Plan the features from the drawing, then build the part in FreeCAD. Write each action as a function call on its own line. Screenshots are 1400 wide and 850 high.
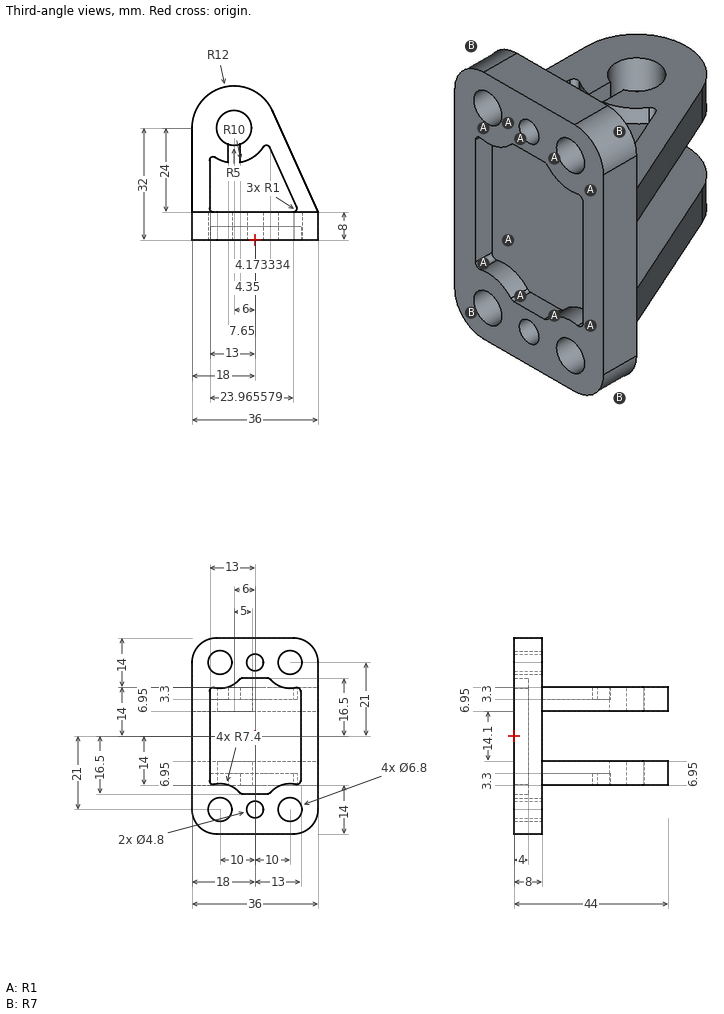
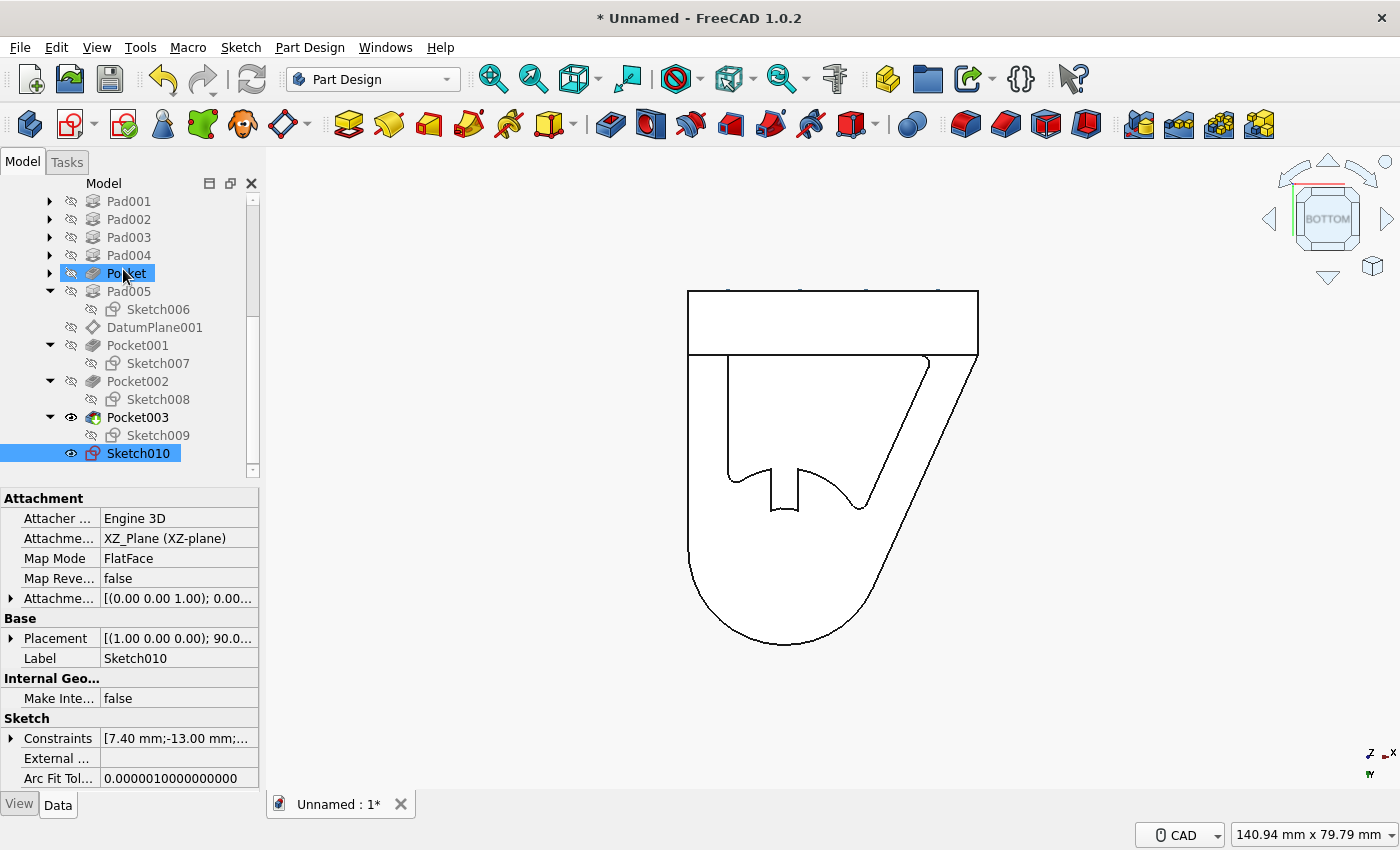
click(612, 124)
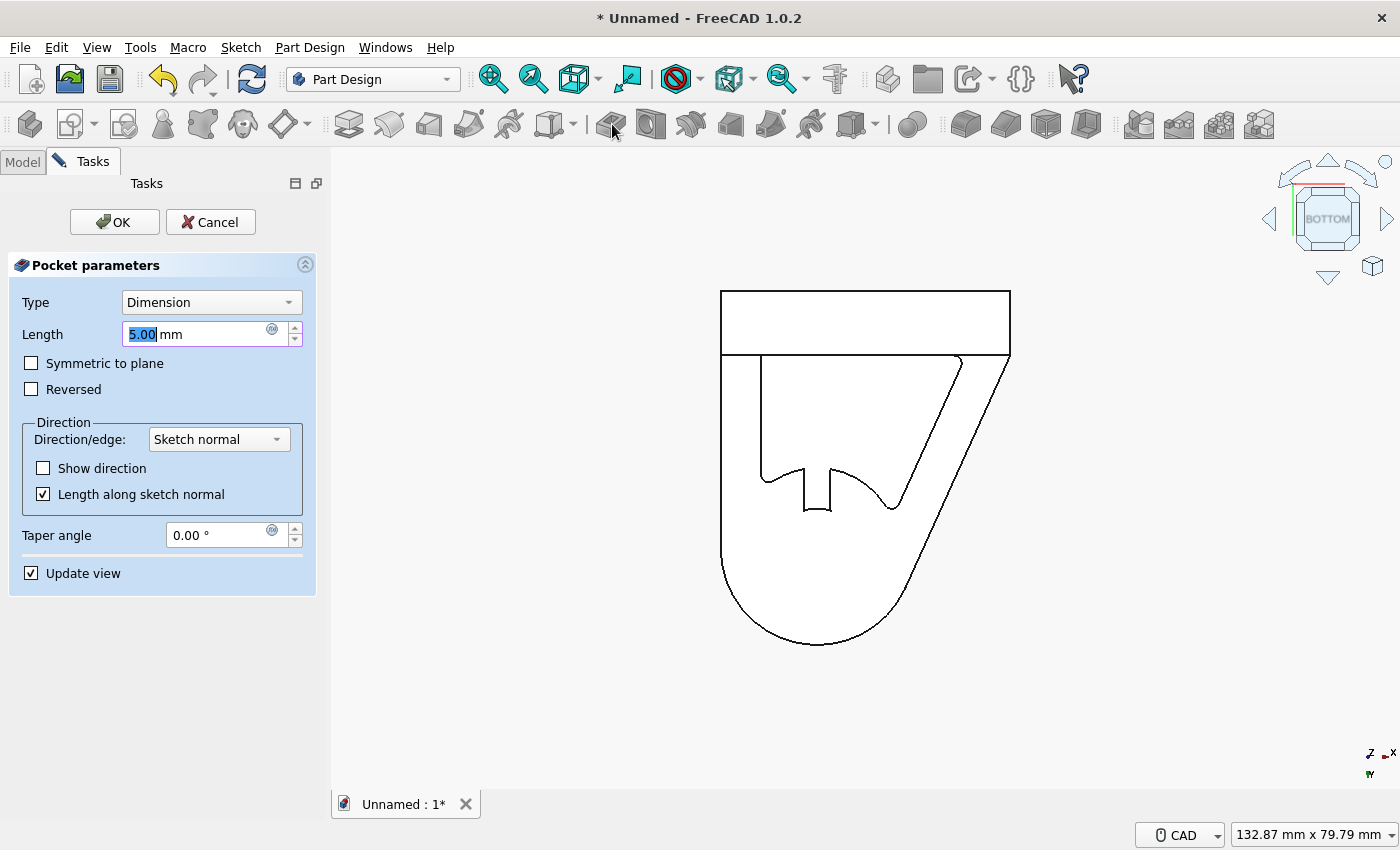
text(4)
key(Tab)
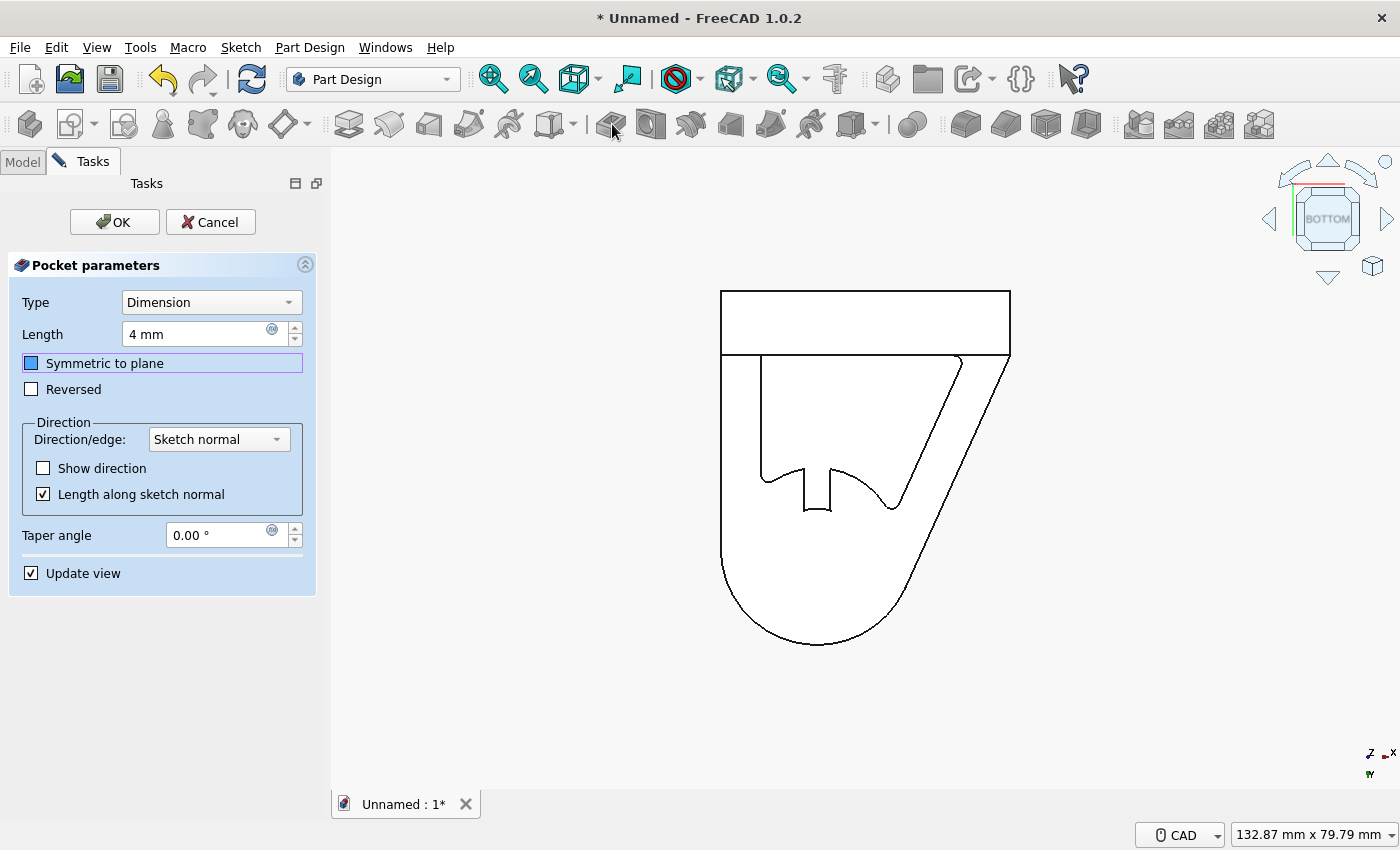
click(115, 222)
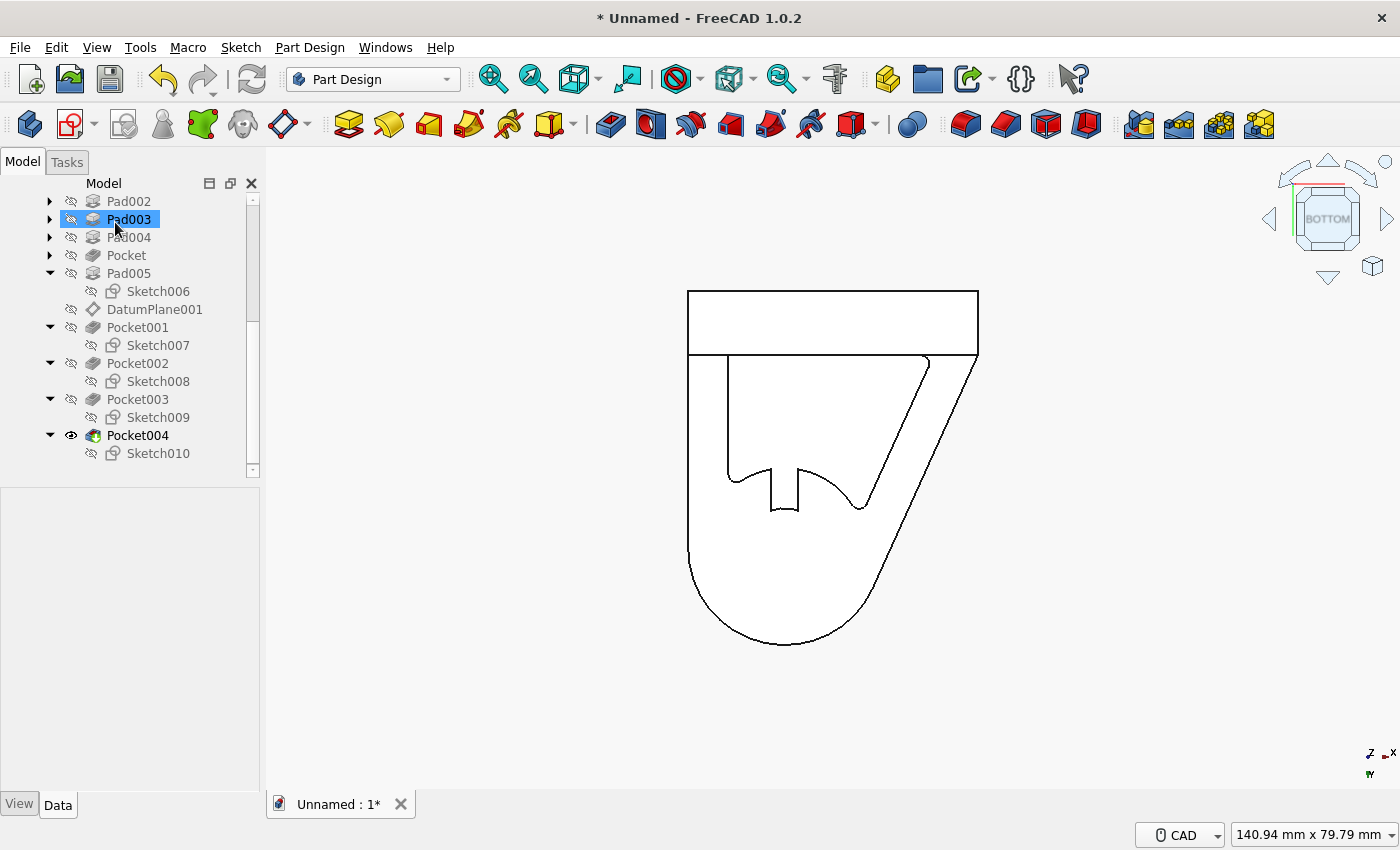
scroll(140, 323, down, 3)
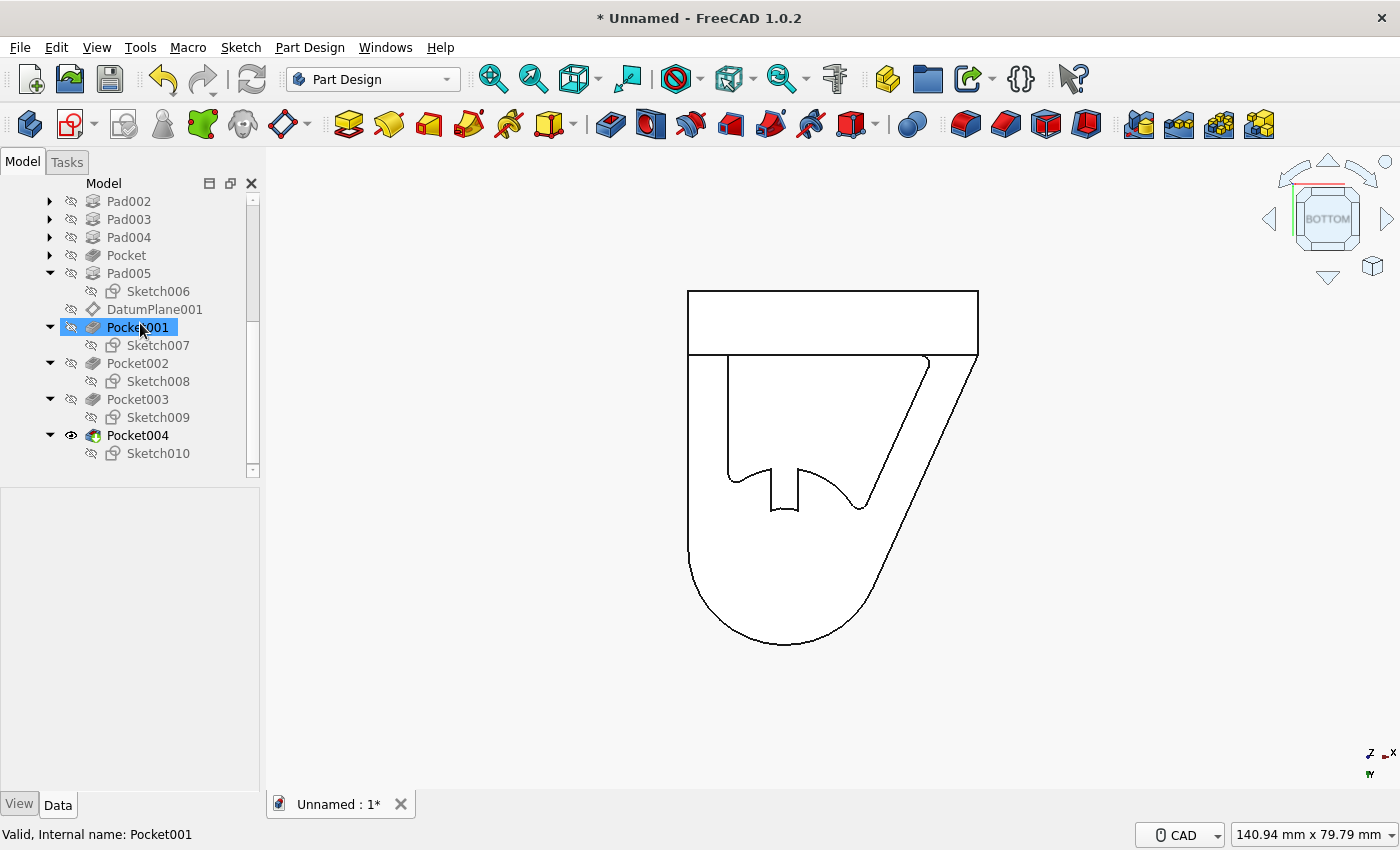
scroll(140, 323, up, 15)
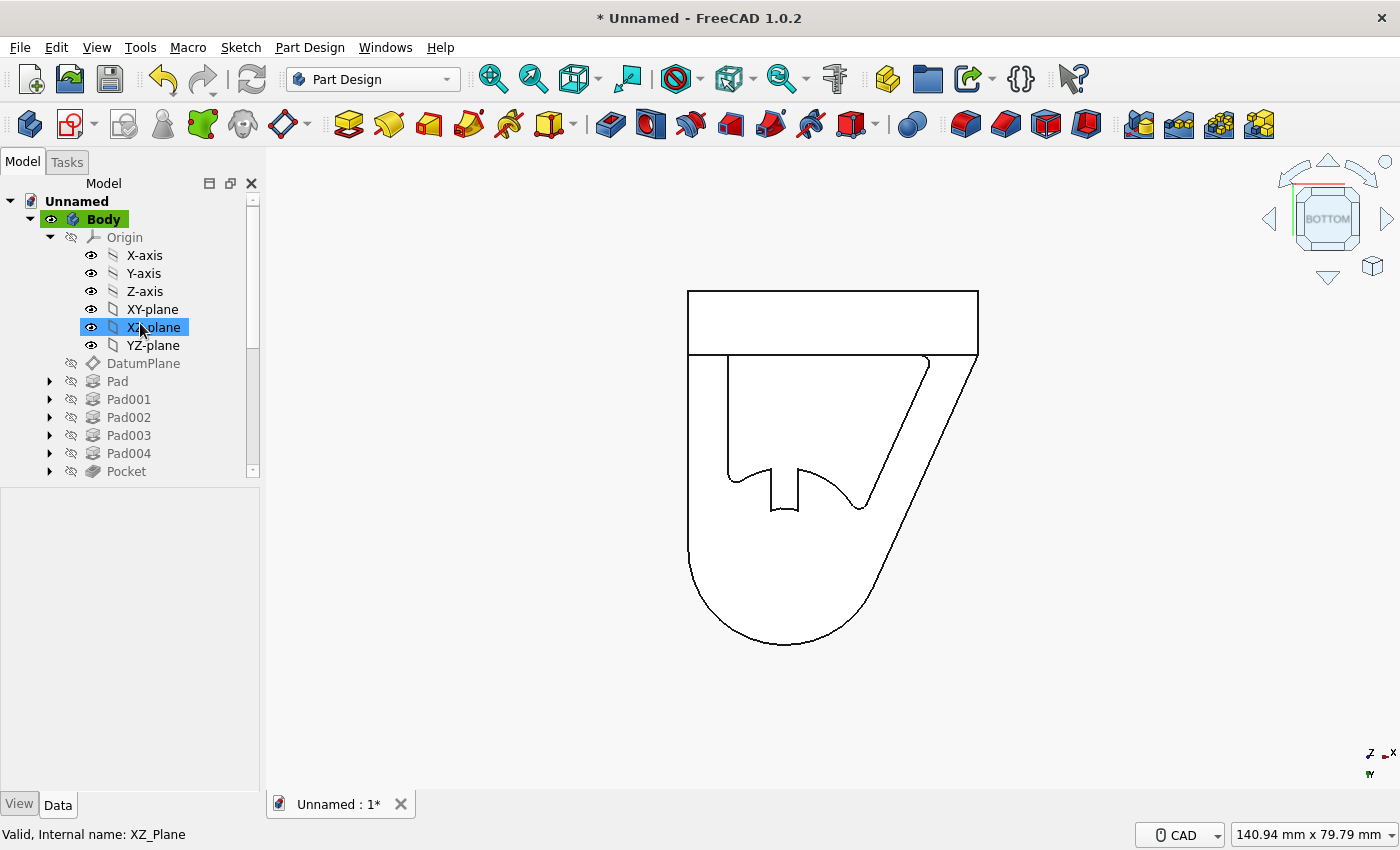
click(136, 327)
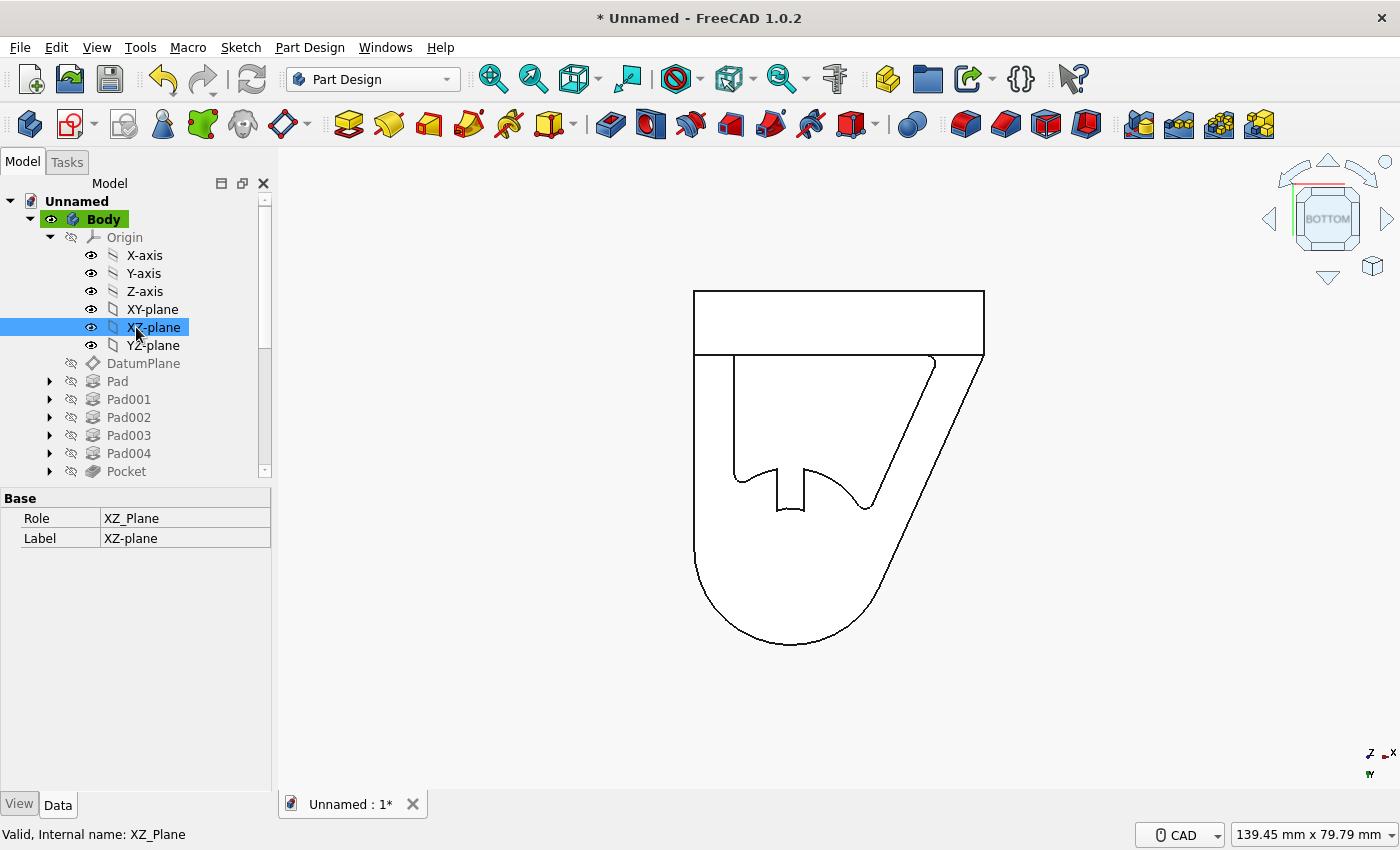
click(284, 124)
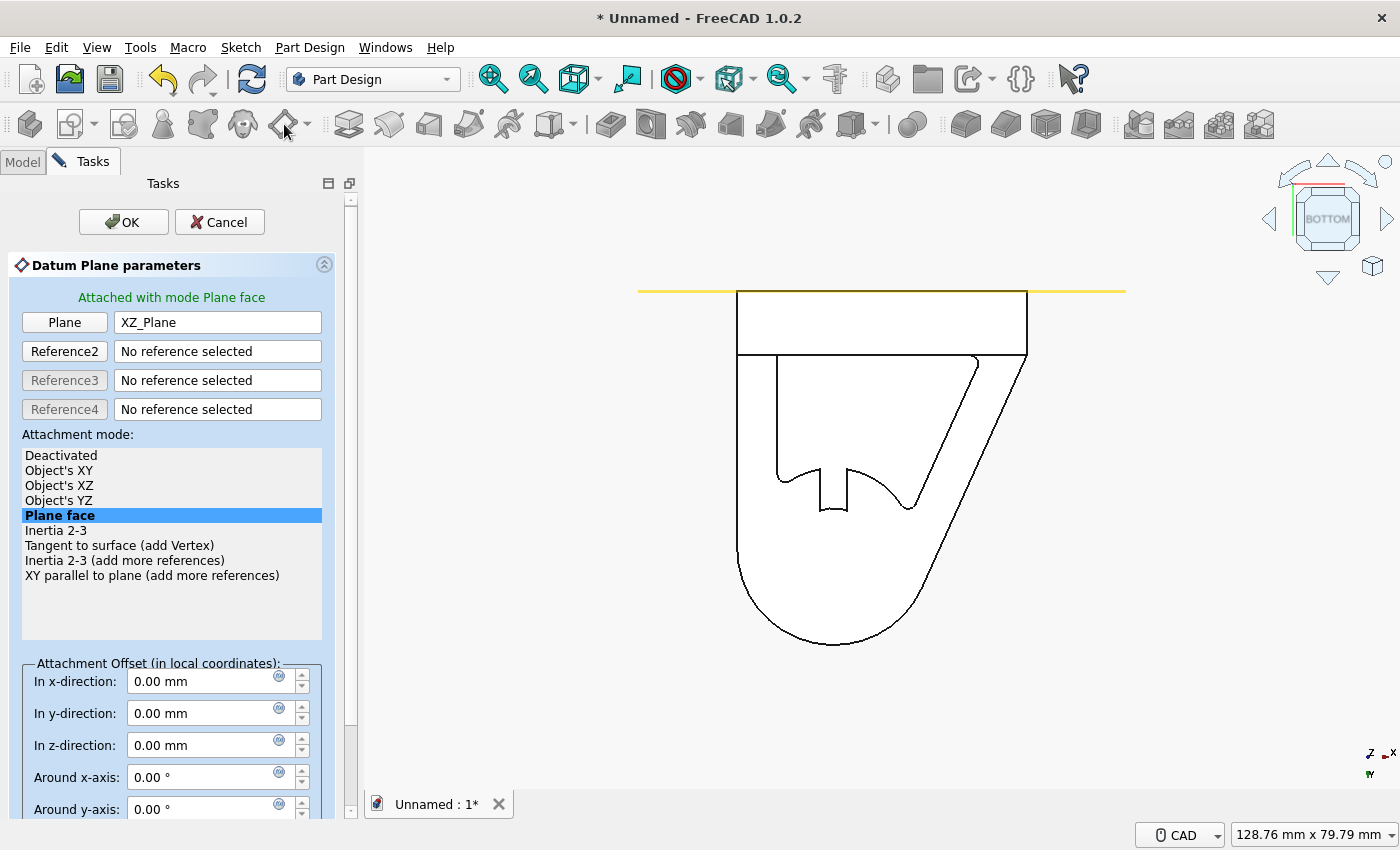
triple_click(210, 745)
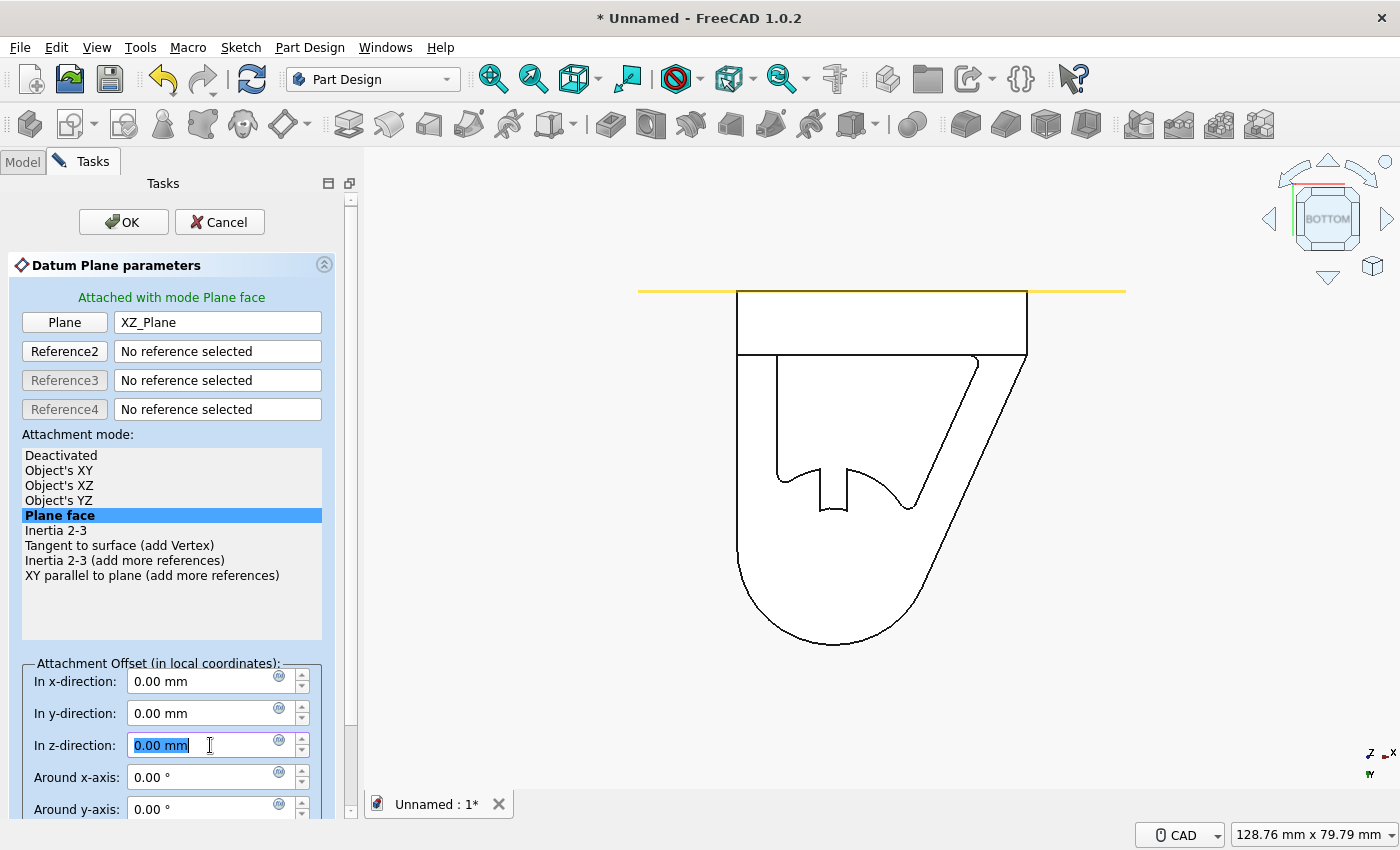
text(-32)
key(Tab)